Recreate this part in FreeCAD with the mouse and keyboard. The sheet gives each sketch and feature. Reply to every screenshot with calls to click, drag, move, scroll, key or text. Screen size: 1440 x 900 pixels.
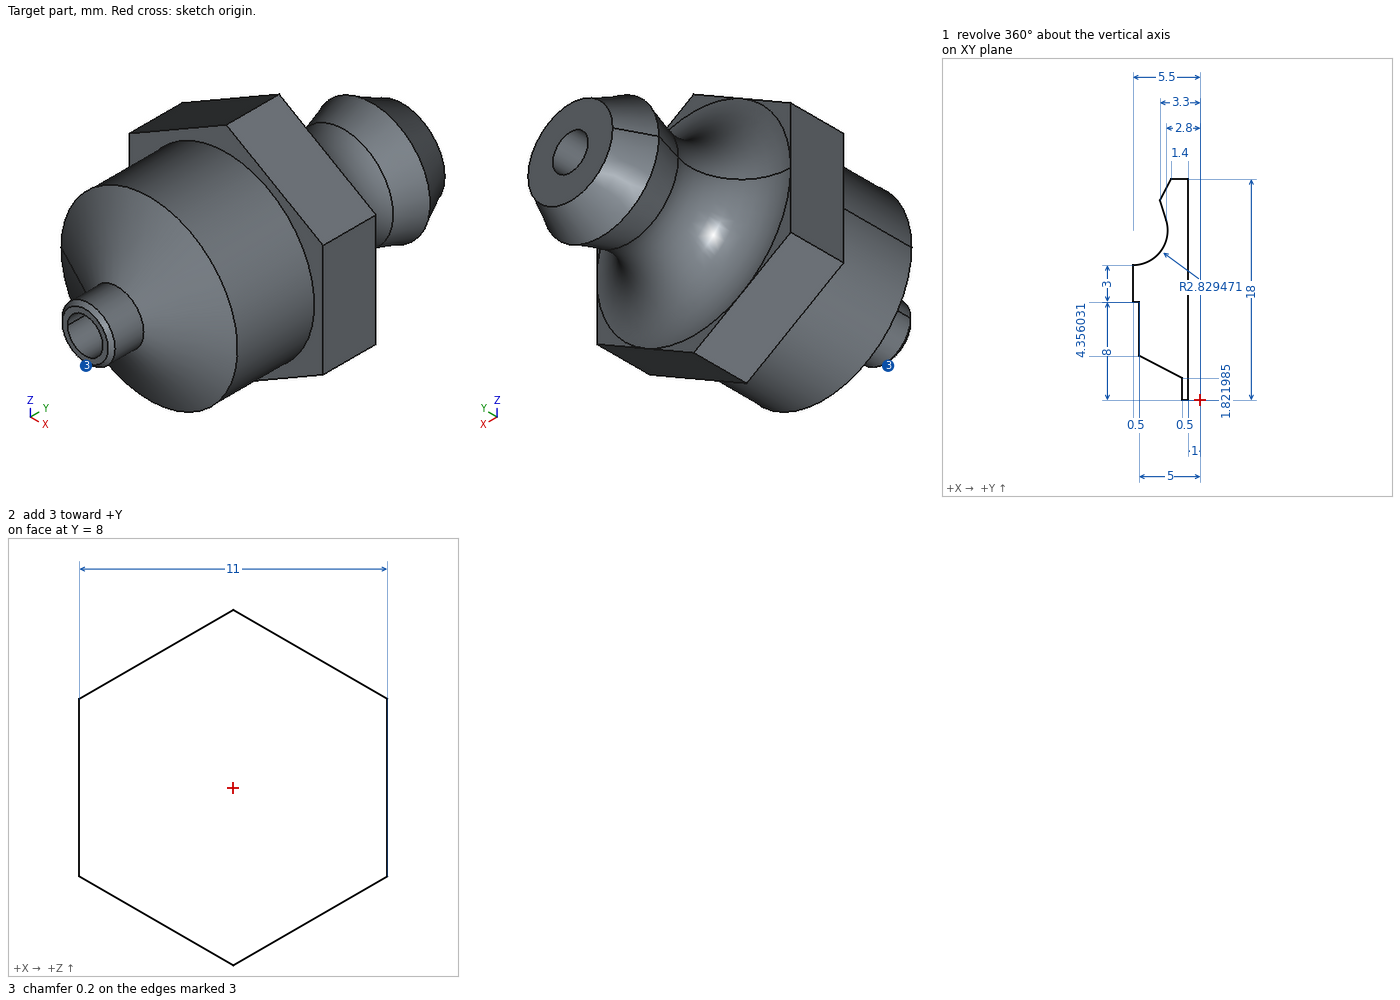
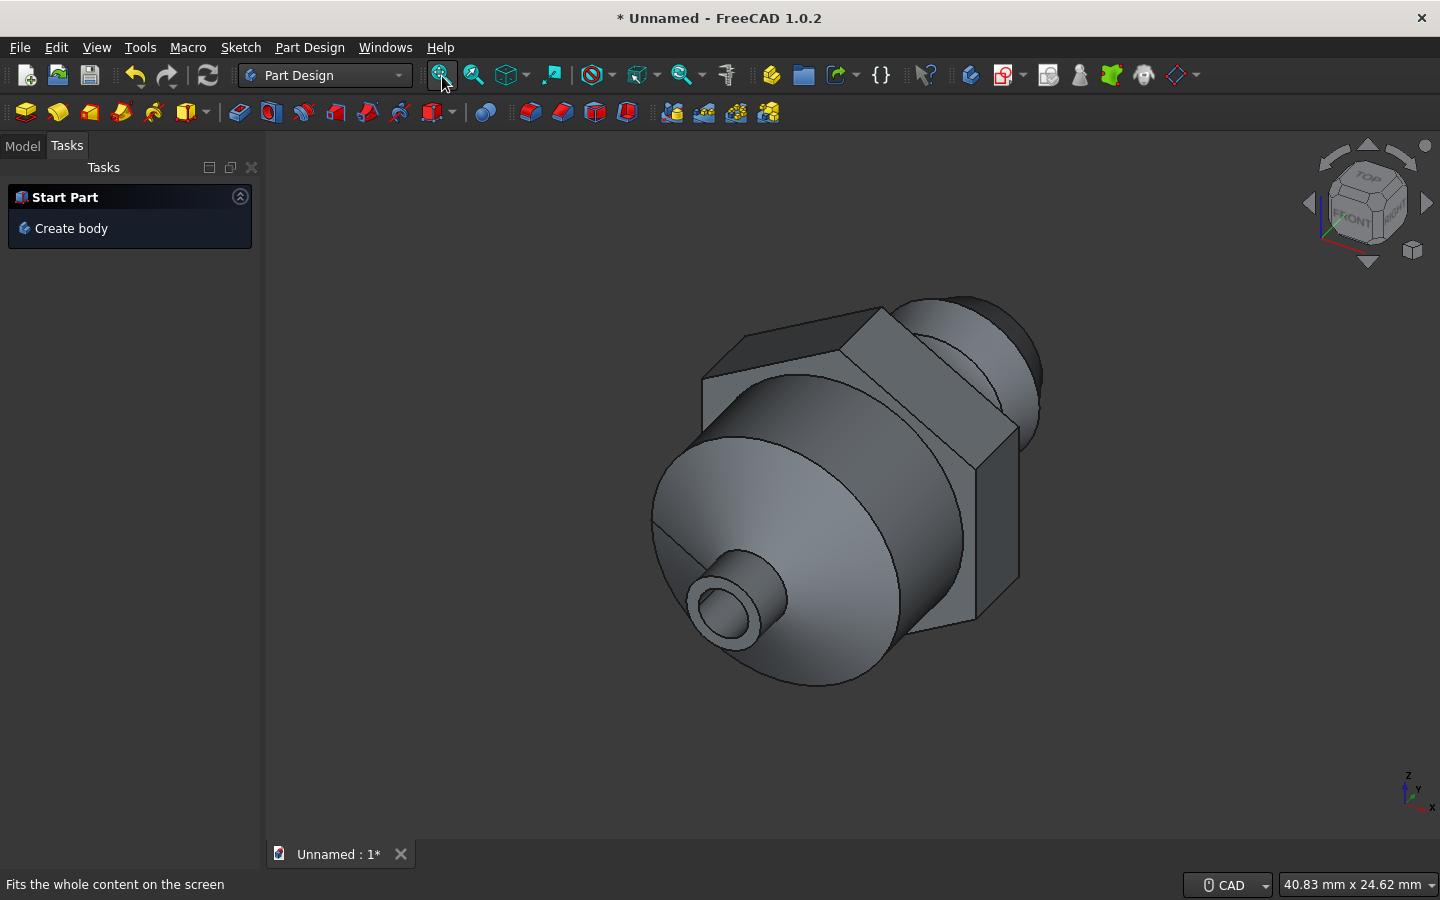
click(761, 625)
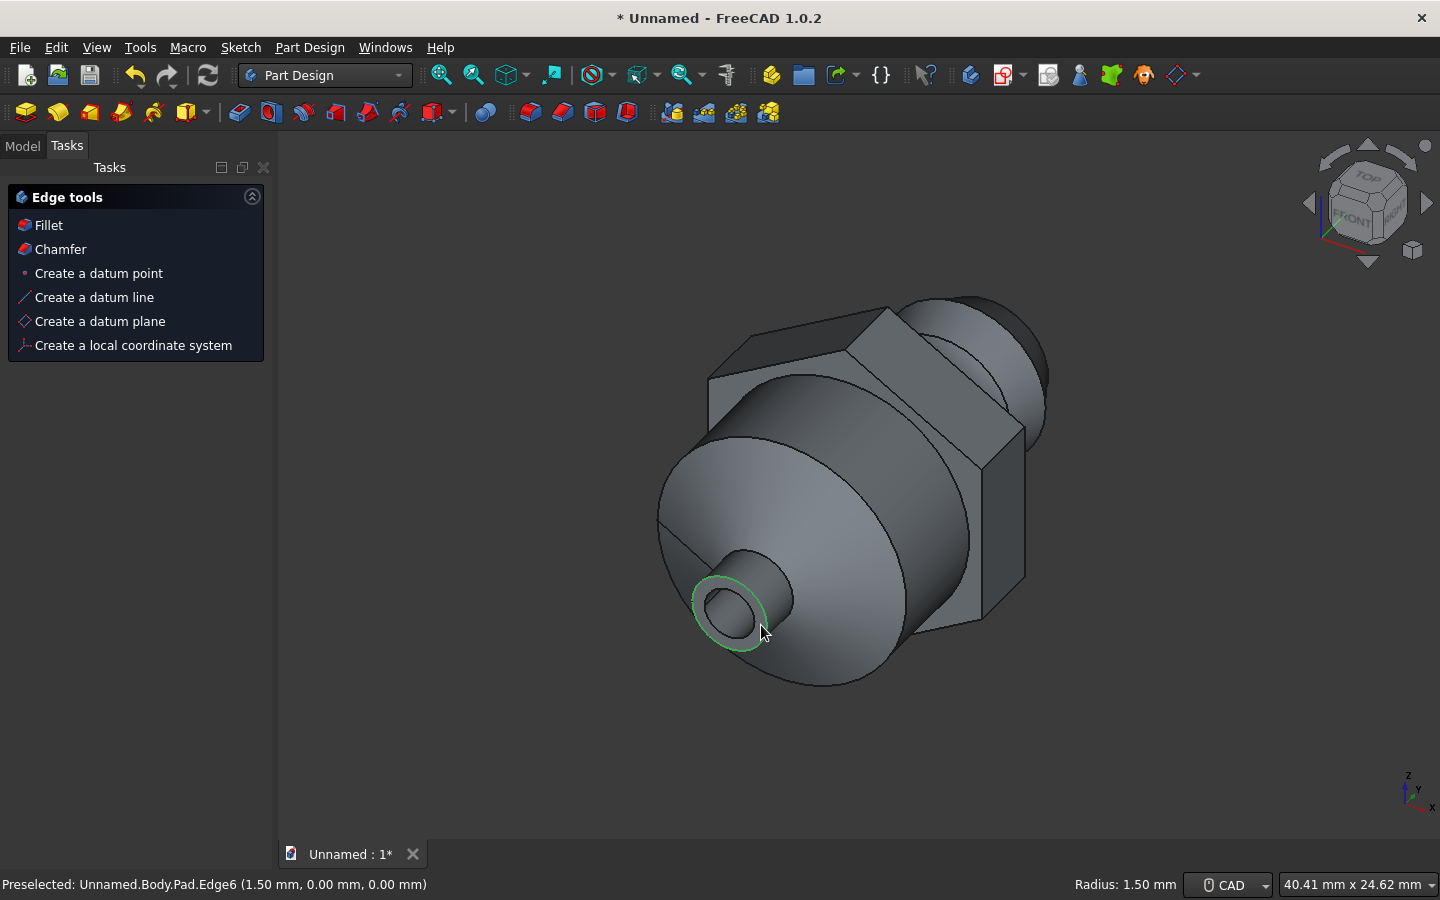
click(564, 112)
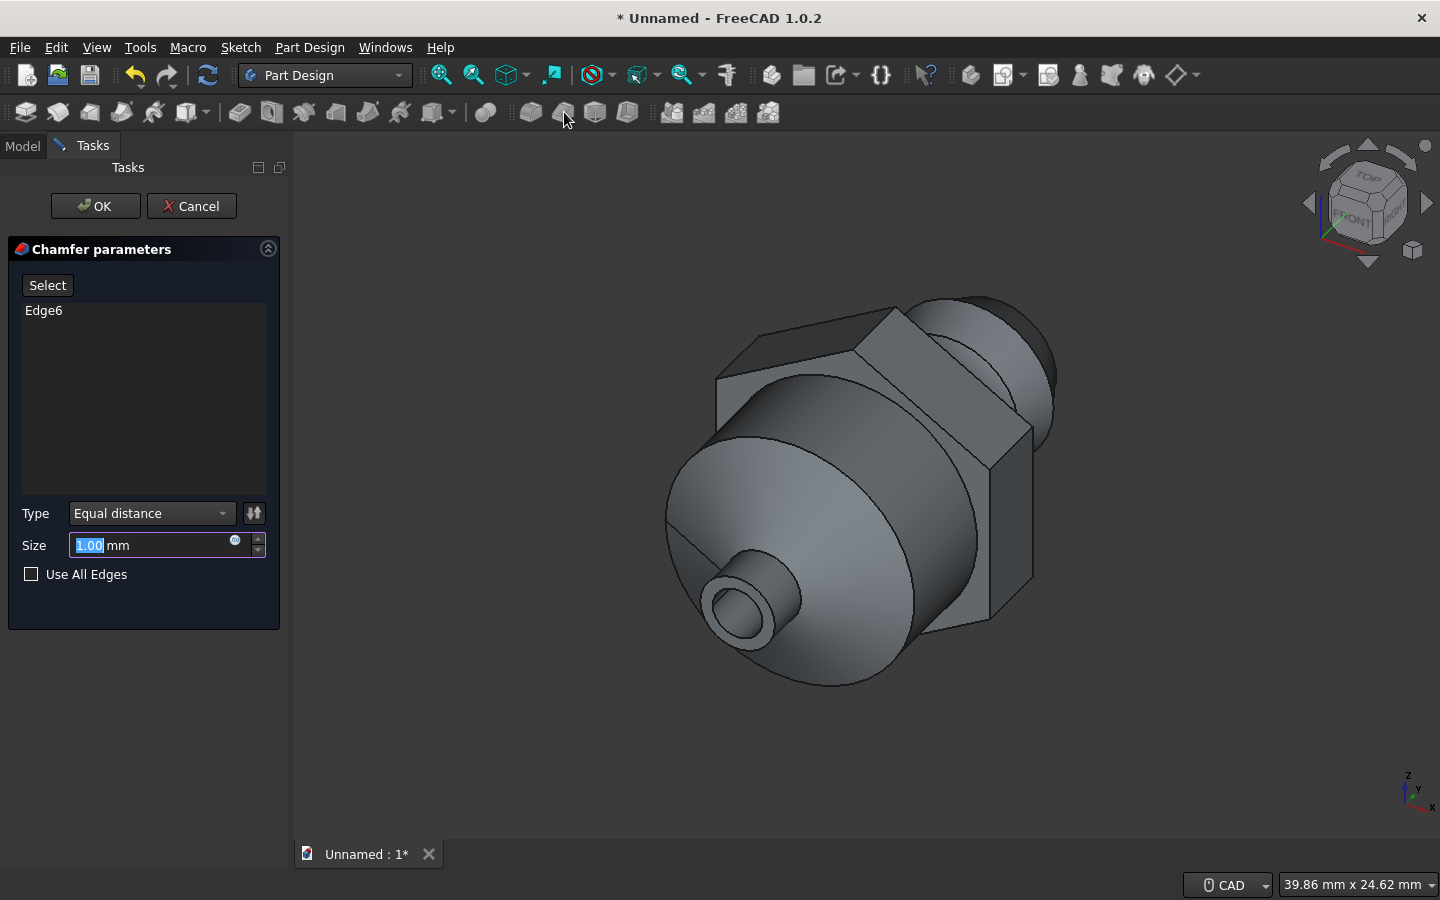
text(0.2)
key(Tab)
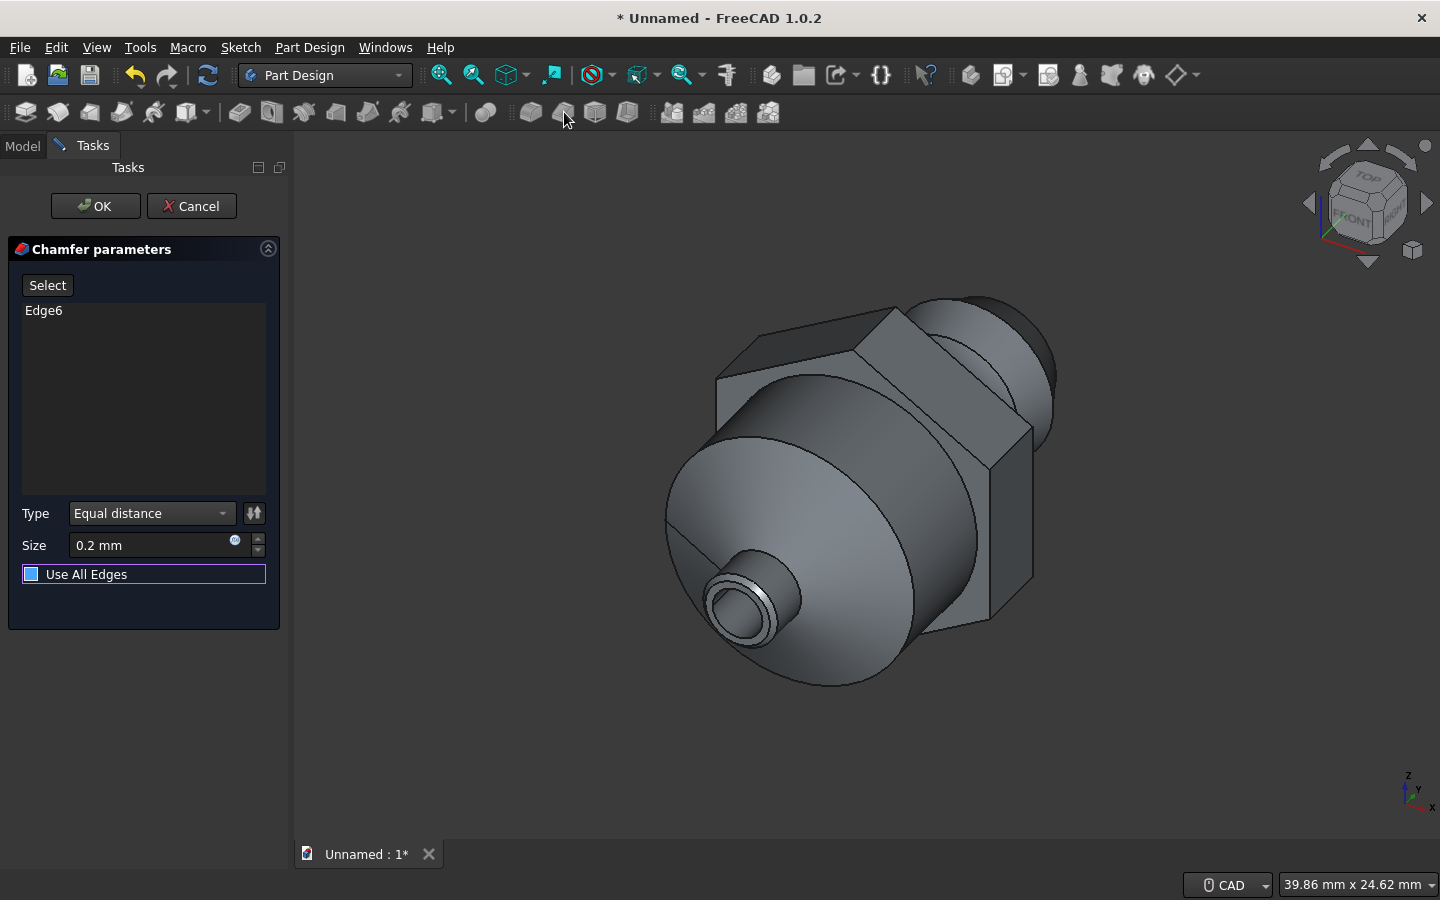
click(96, 206)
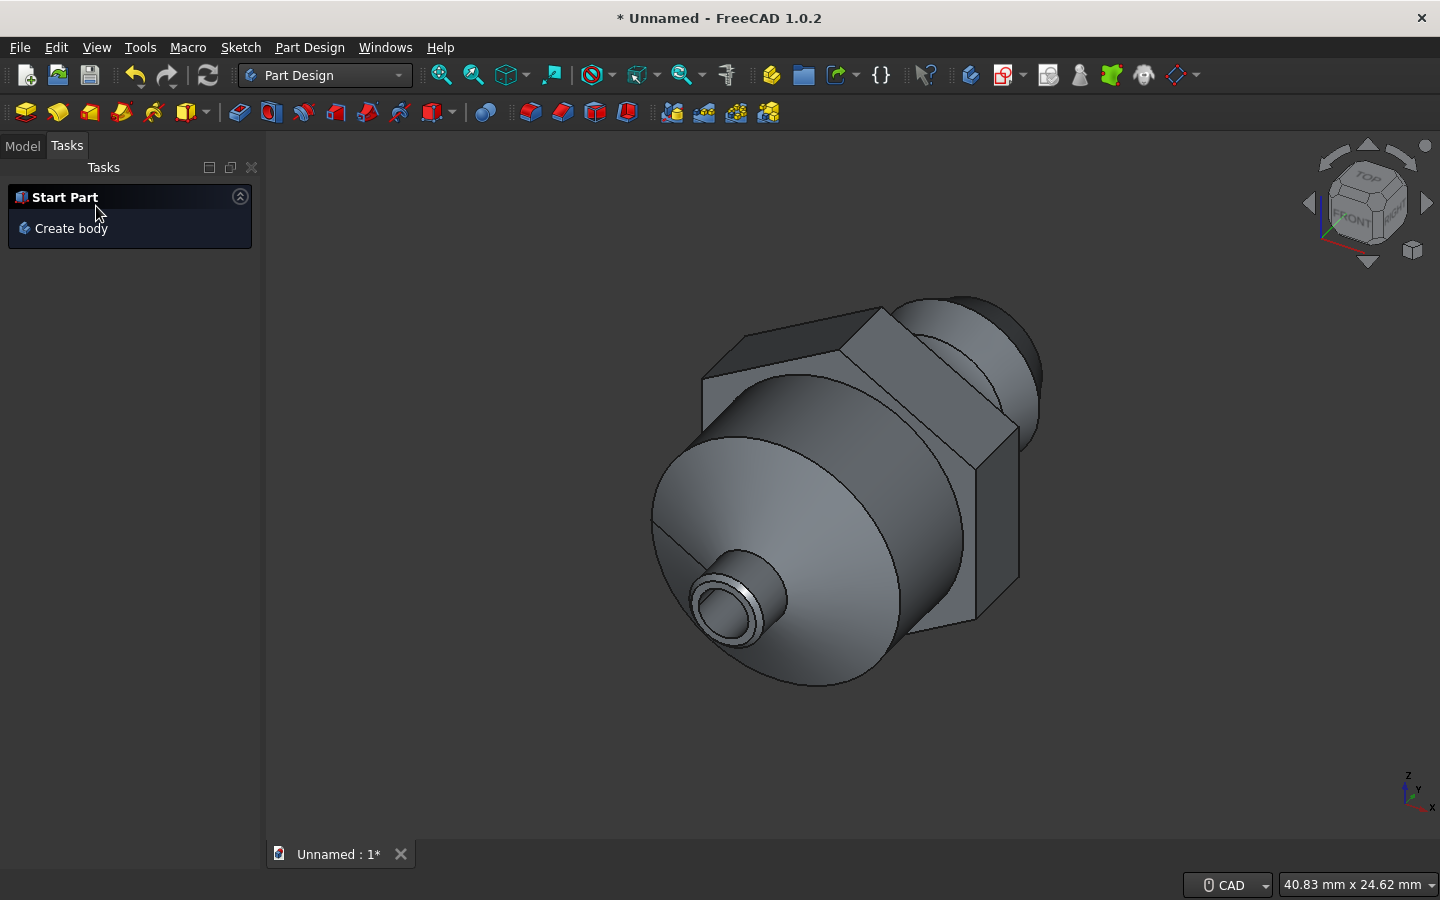
key(0)